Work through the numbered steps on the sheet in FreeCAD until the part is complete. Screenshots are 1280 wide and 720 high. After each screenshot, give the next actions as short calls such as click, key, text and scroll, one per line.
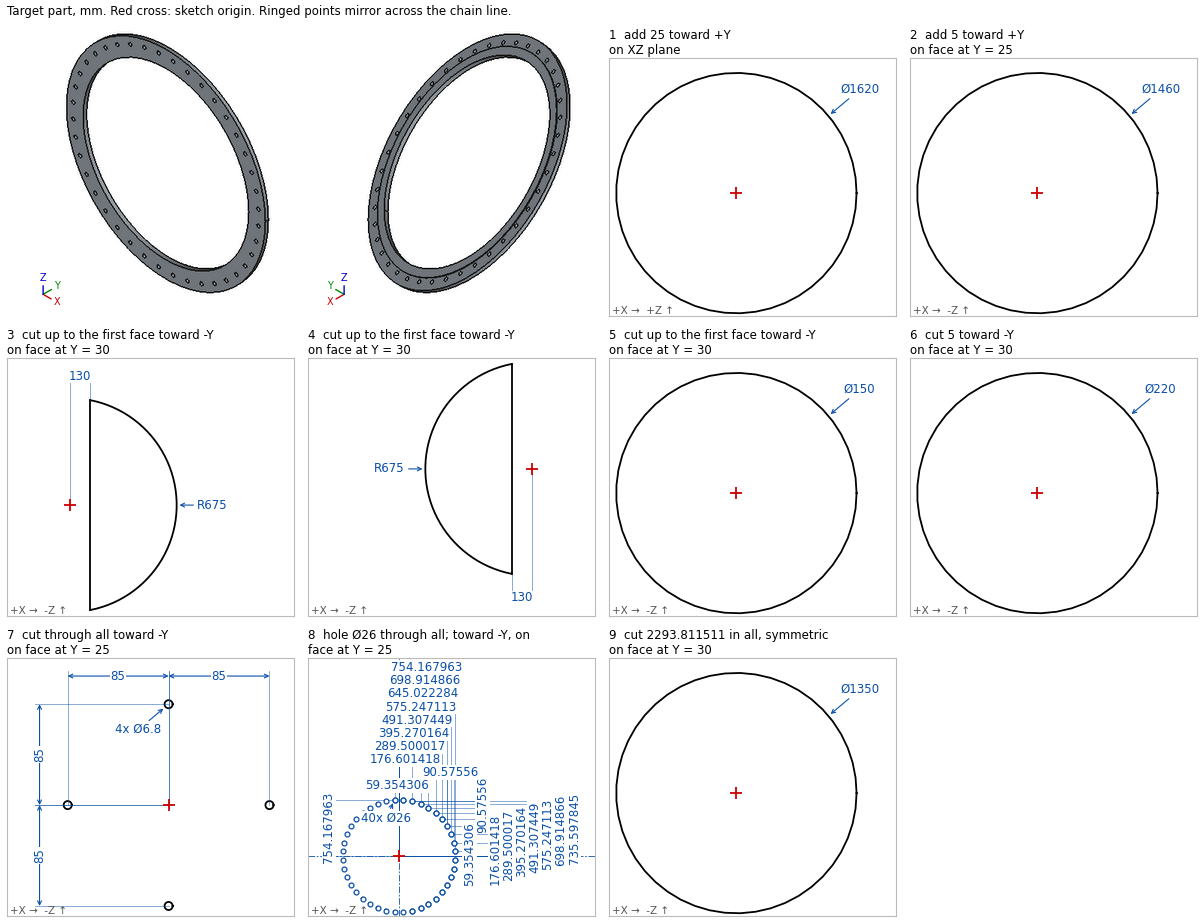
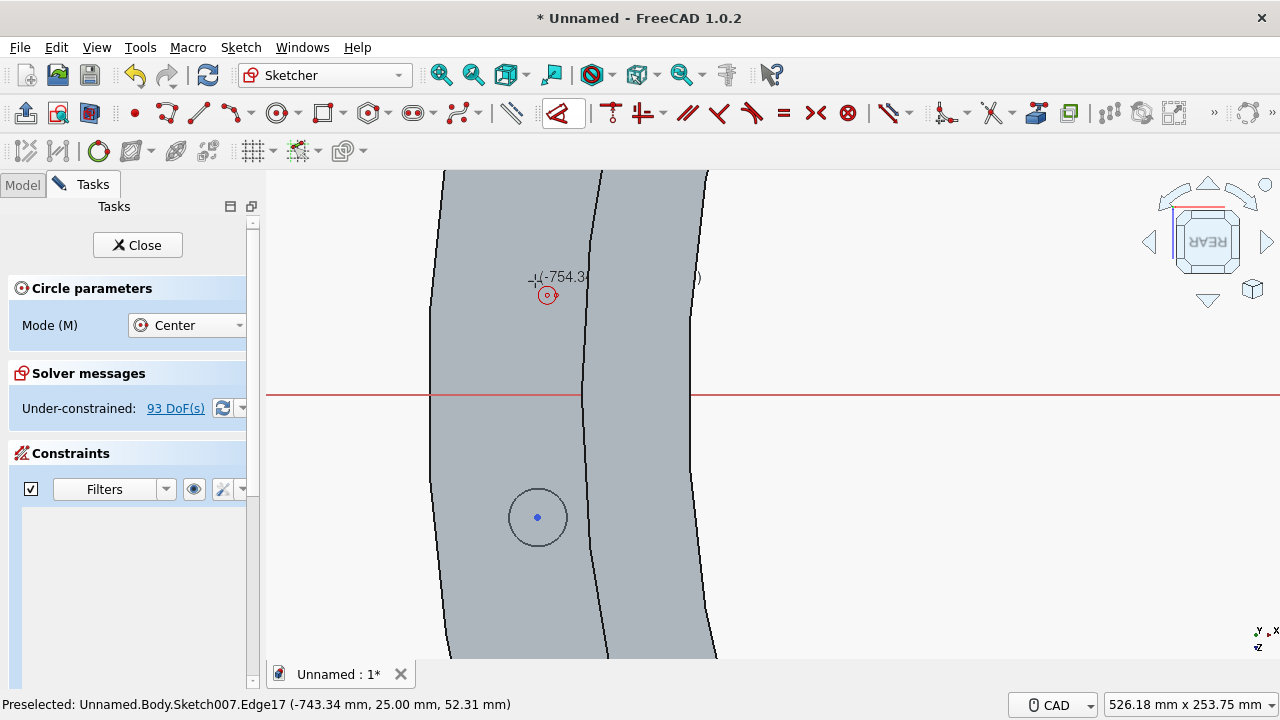
scroll(544, 417, down, 11)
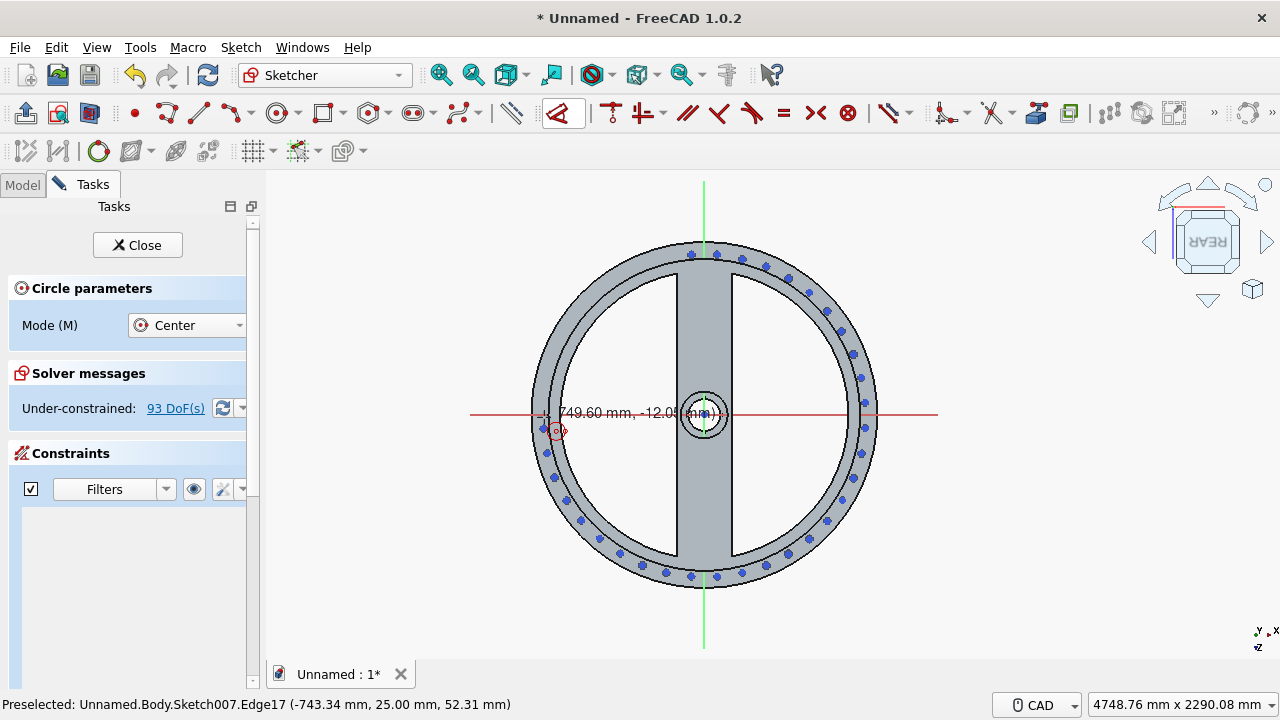
scroll(543, 402, up, 2)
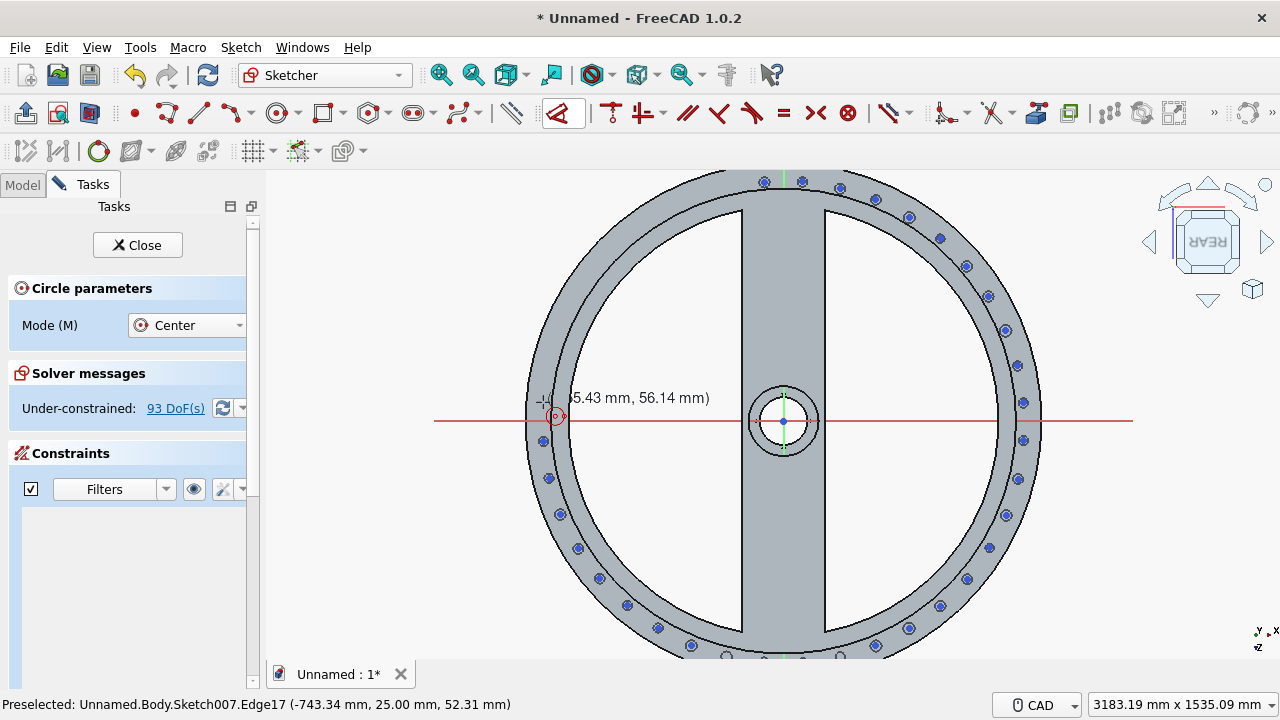
click(543, 402)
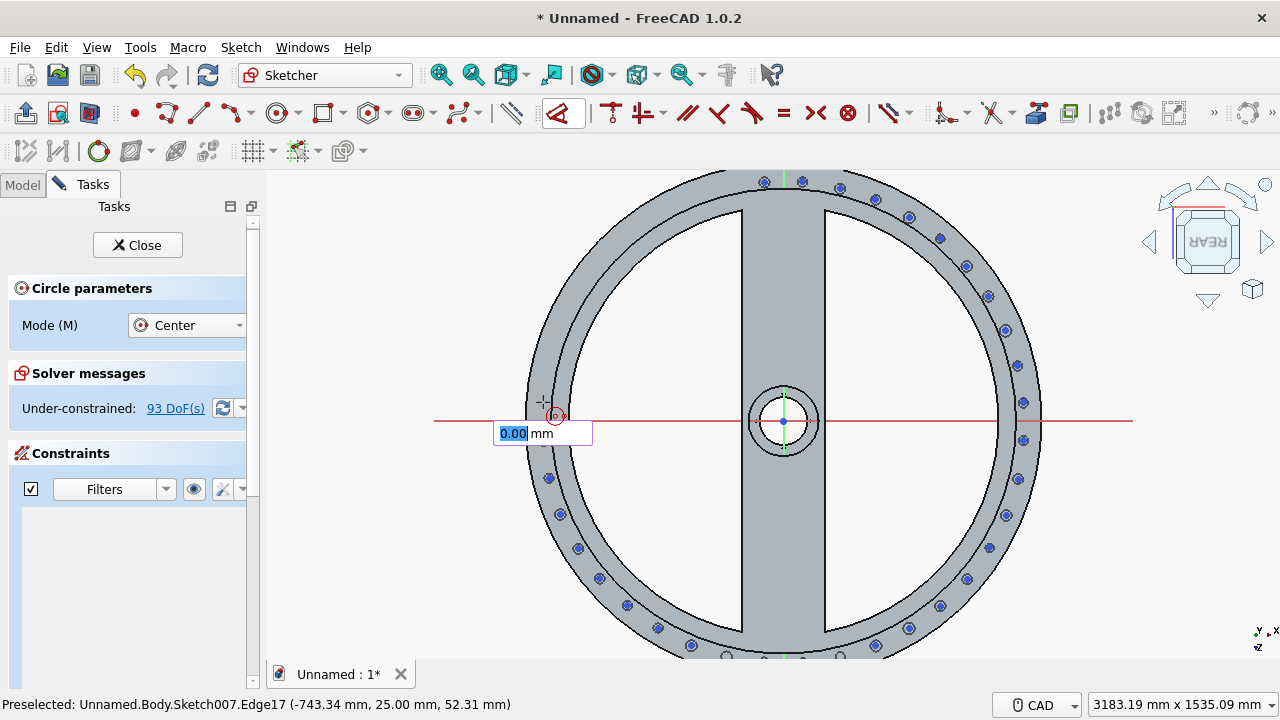
scroll(546, 399, up, 7)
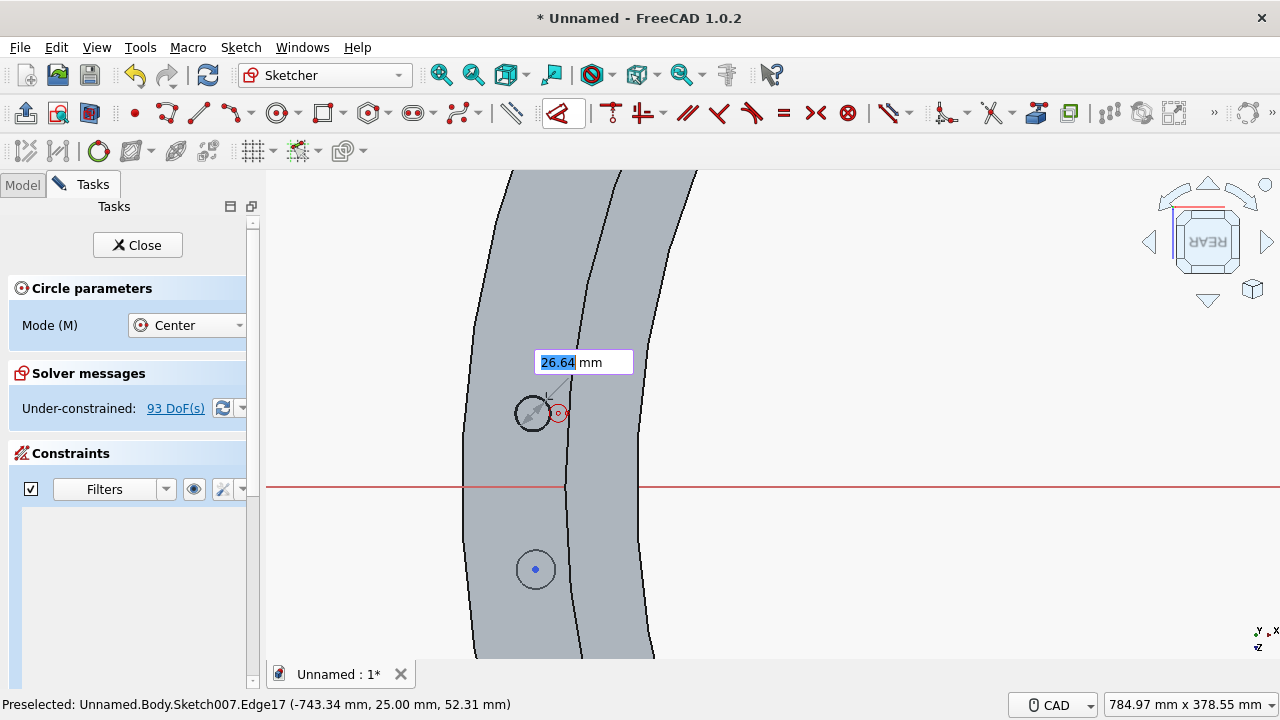
click(546, 399)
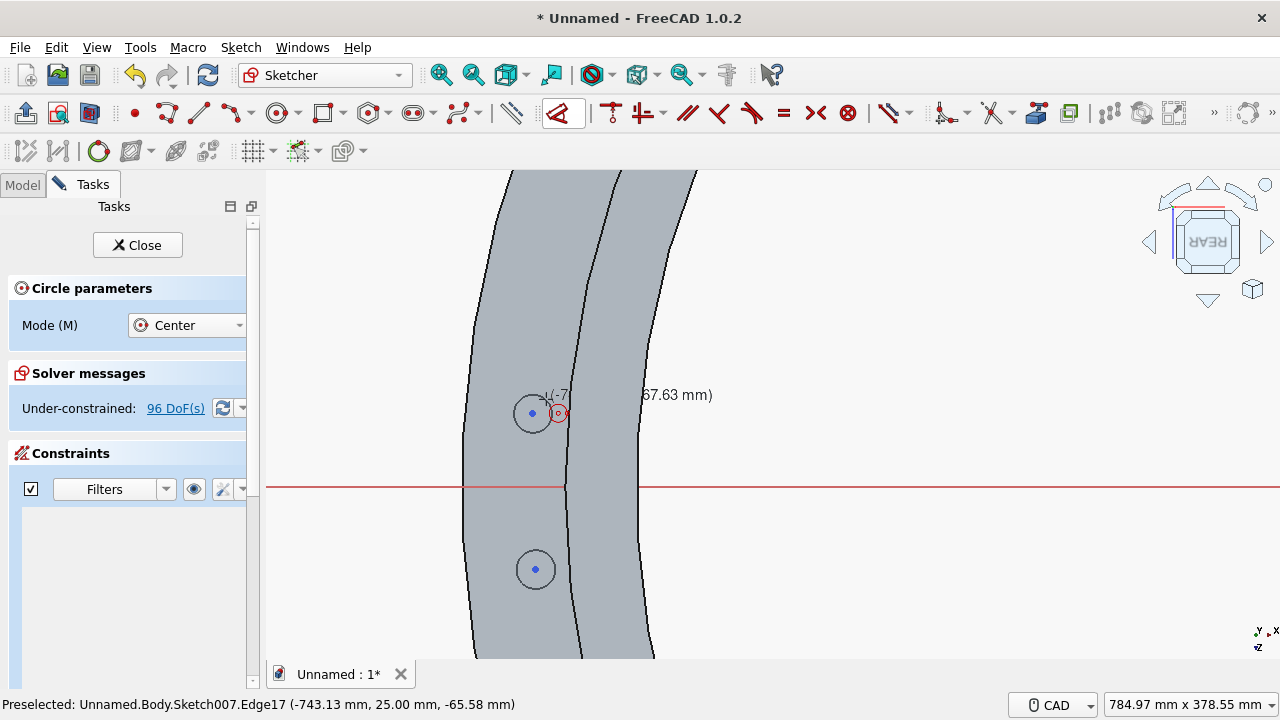
scroll(558, 259, up, 2)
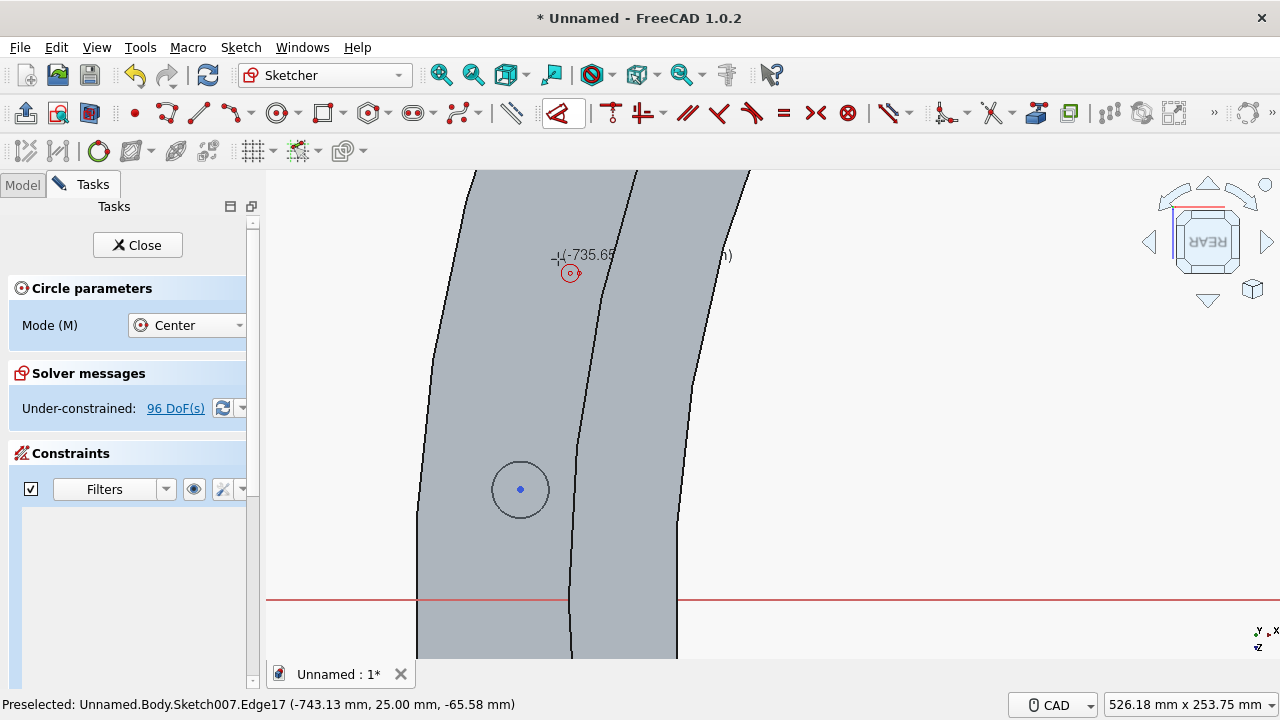
scroll(546, 391, down, 11)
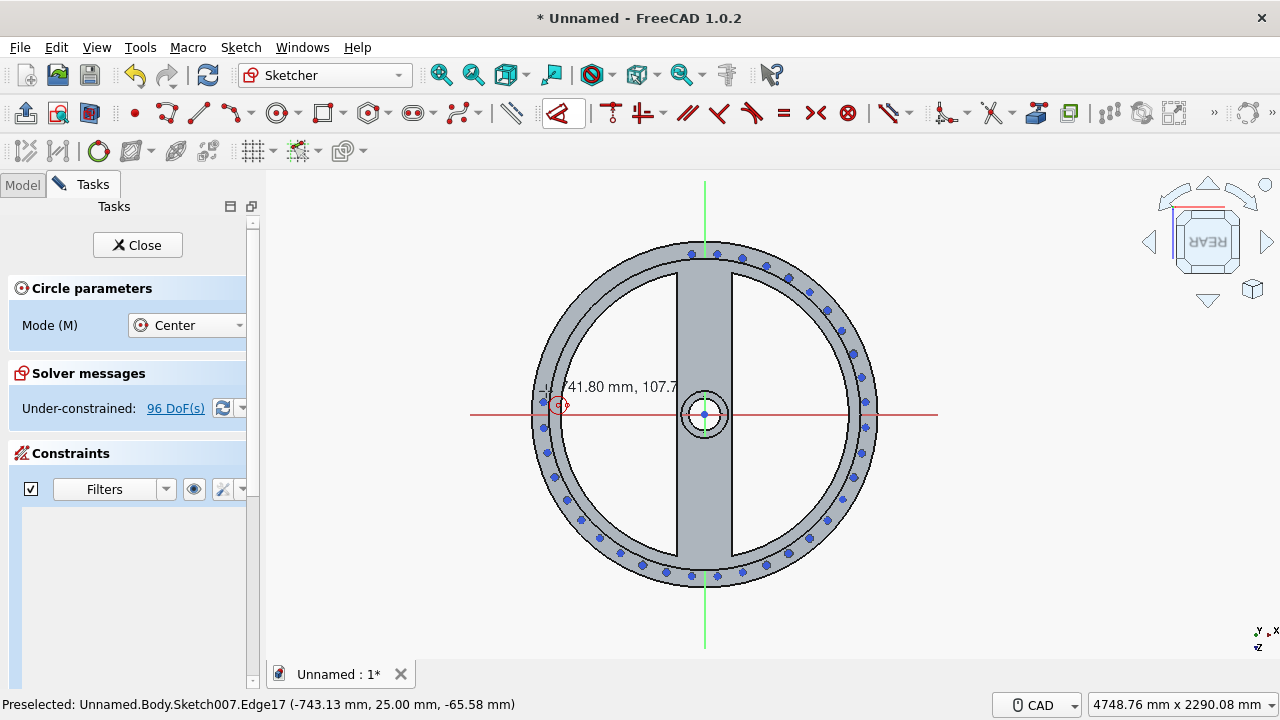
click(548, 377)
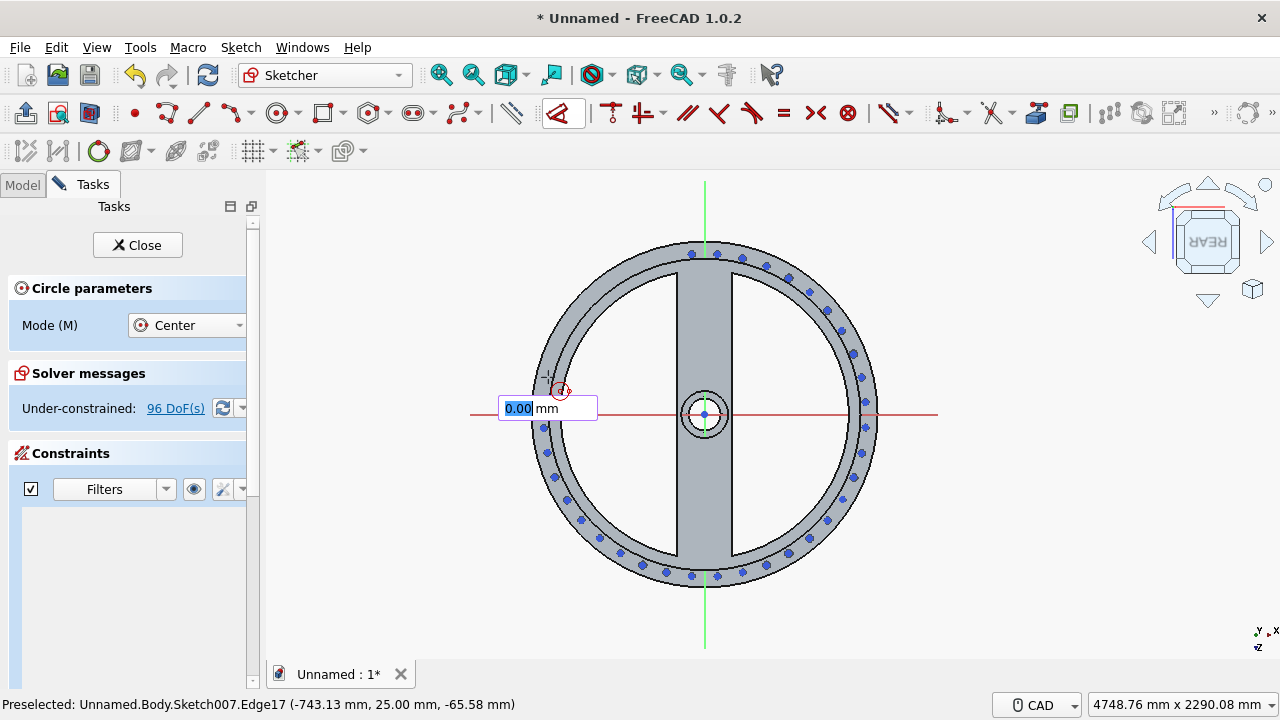
scroll(550, 375, up, 9)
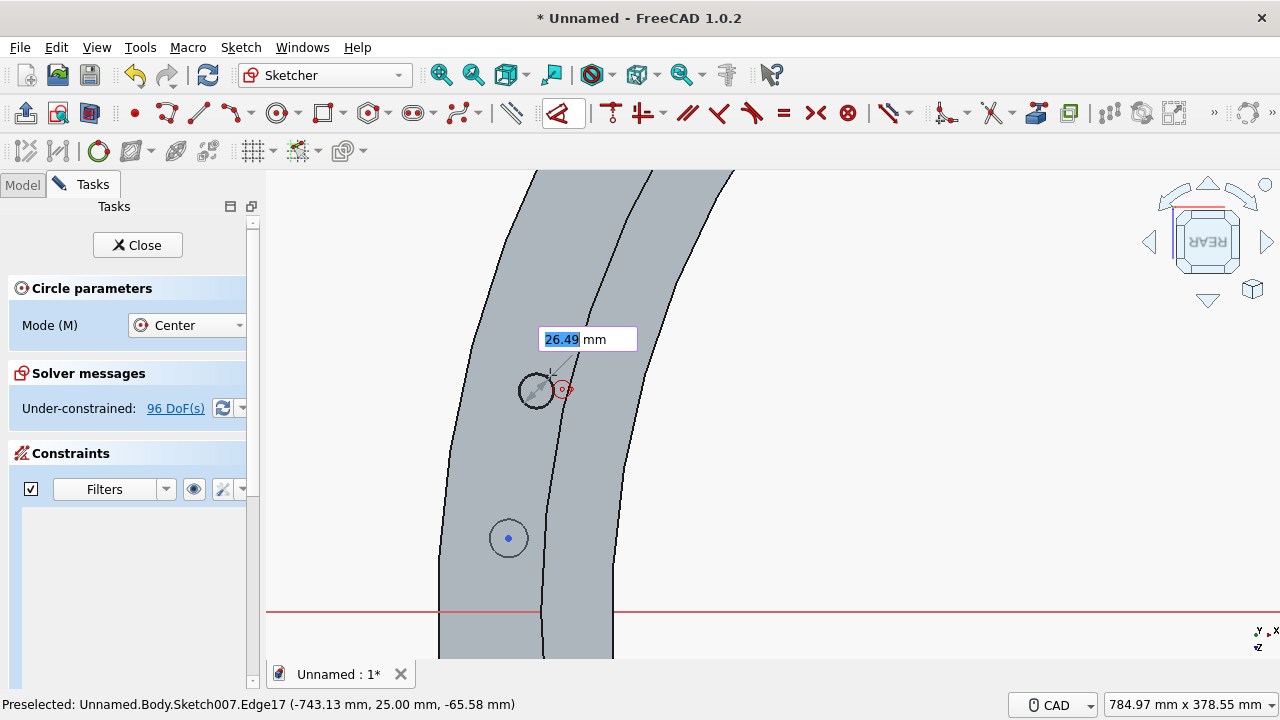
click(546, 372)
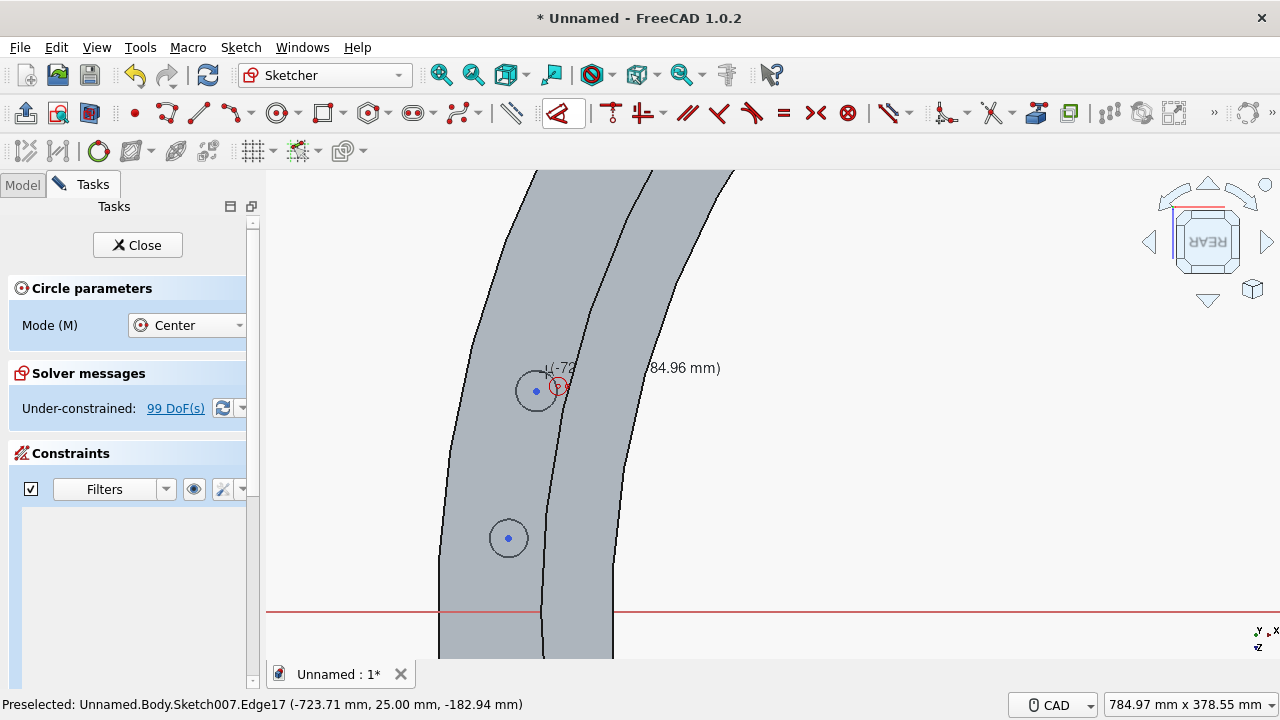
scroll(581, 238, up, 2)